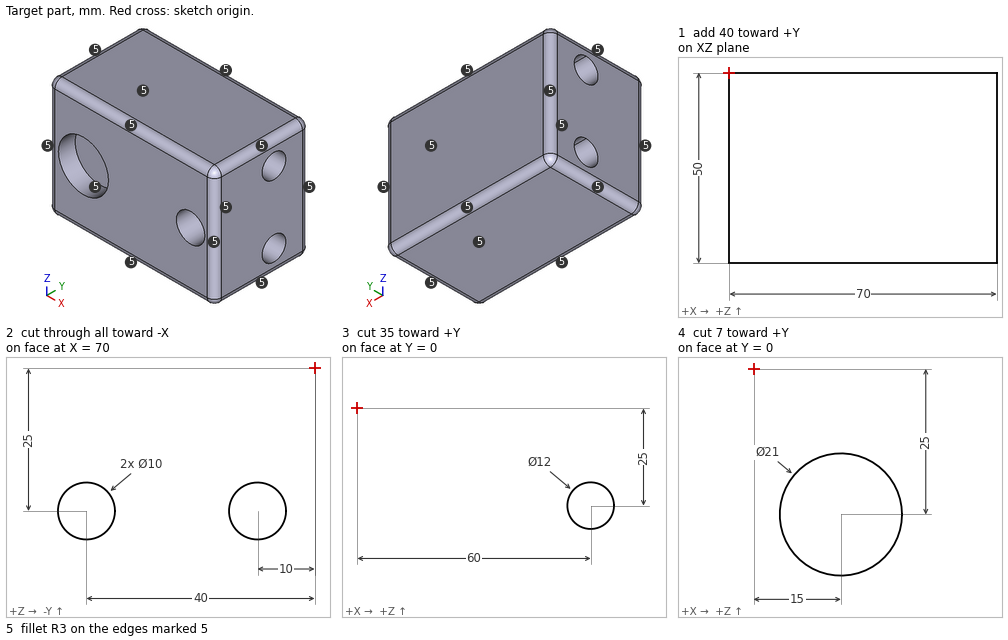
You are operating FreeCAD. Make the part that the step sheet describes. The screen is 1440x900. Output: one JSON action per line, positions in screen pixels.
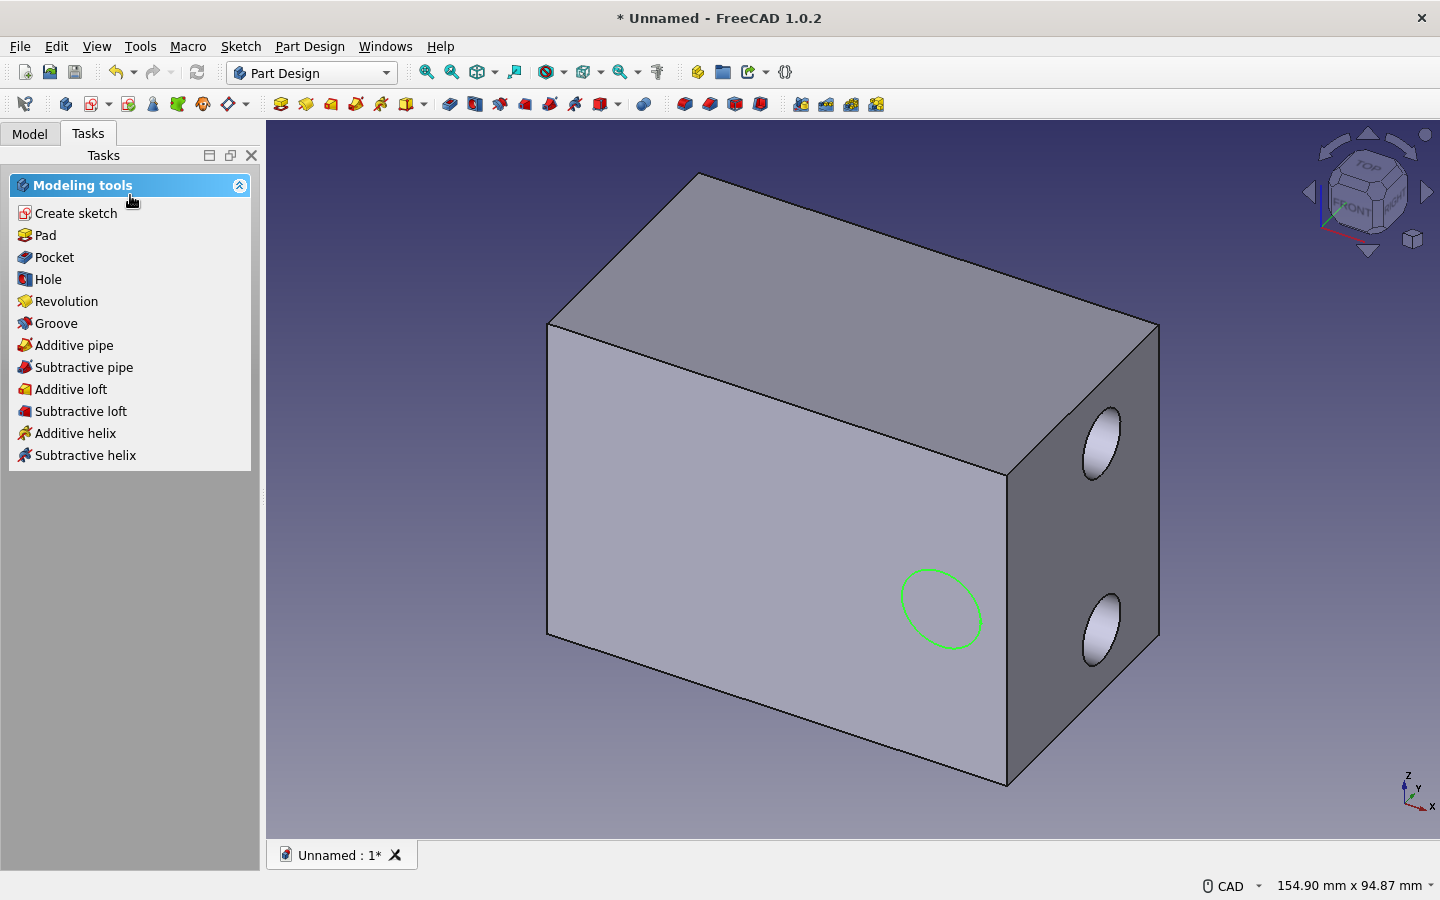
{"action": "left_click", "coordinate": [450, 104]}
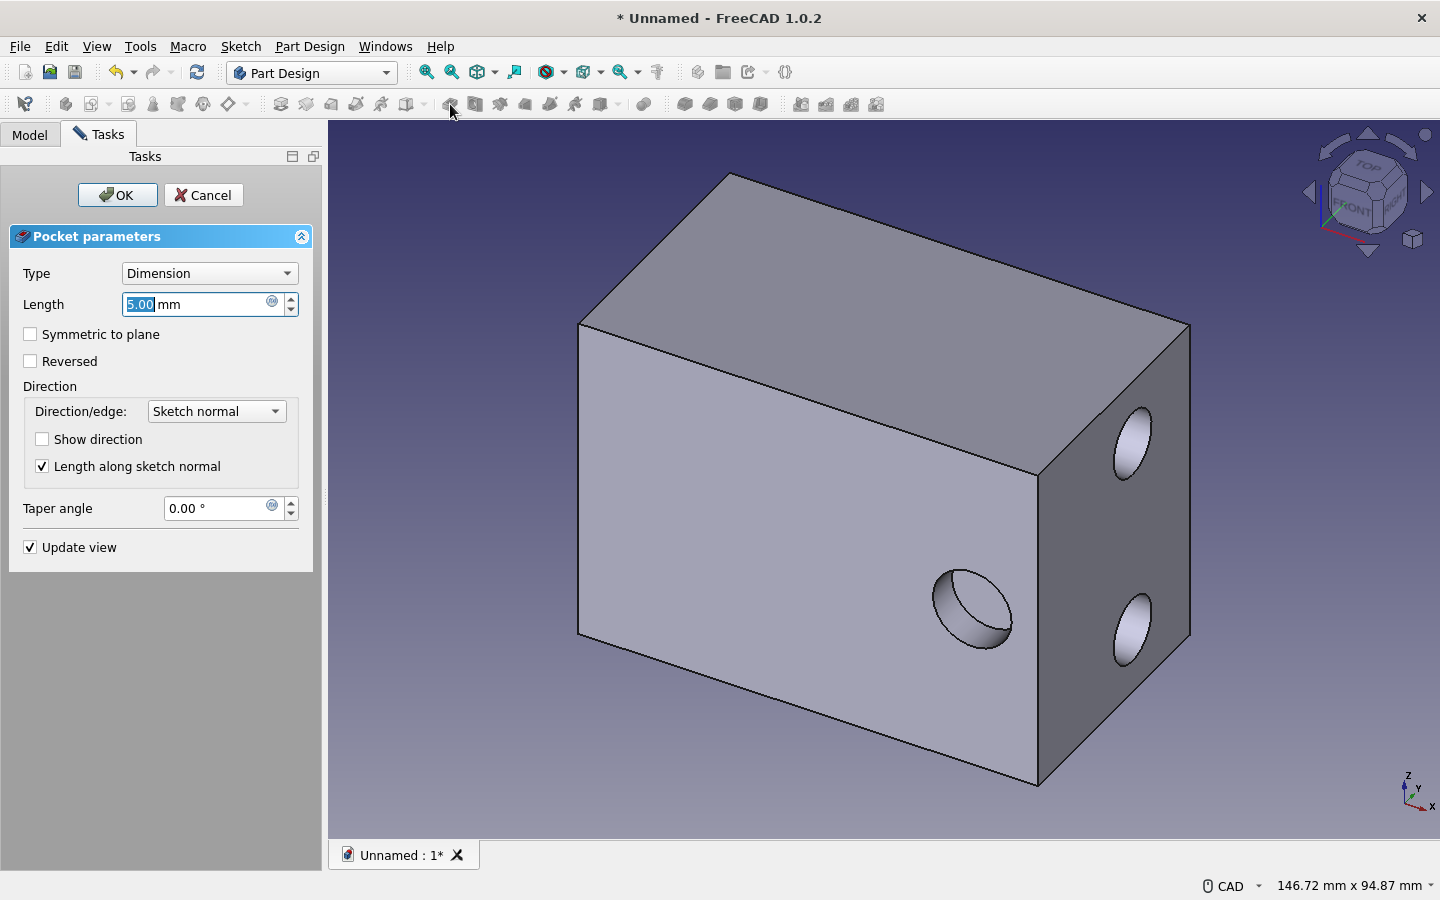
{"action": "type", "text": "35"}
{"action": "key", "text": "Tab"}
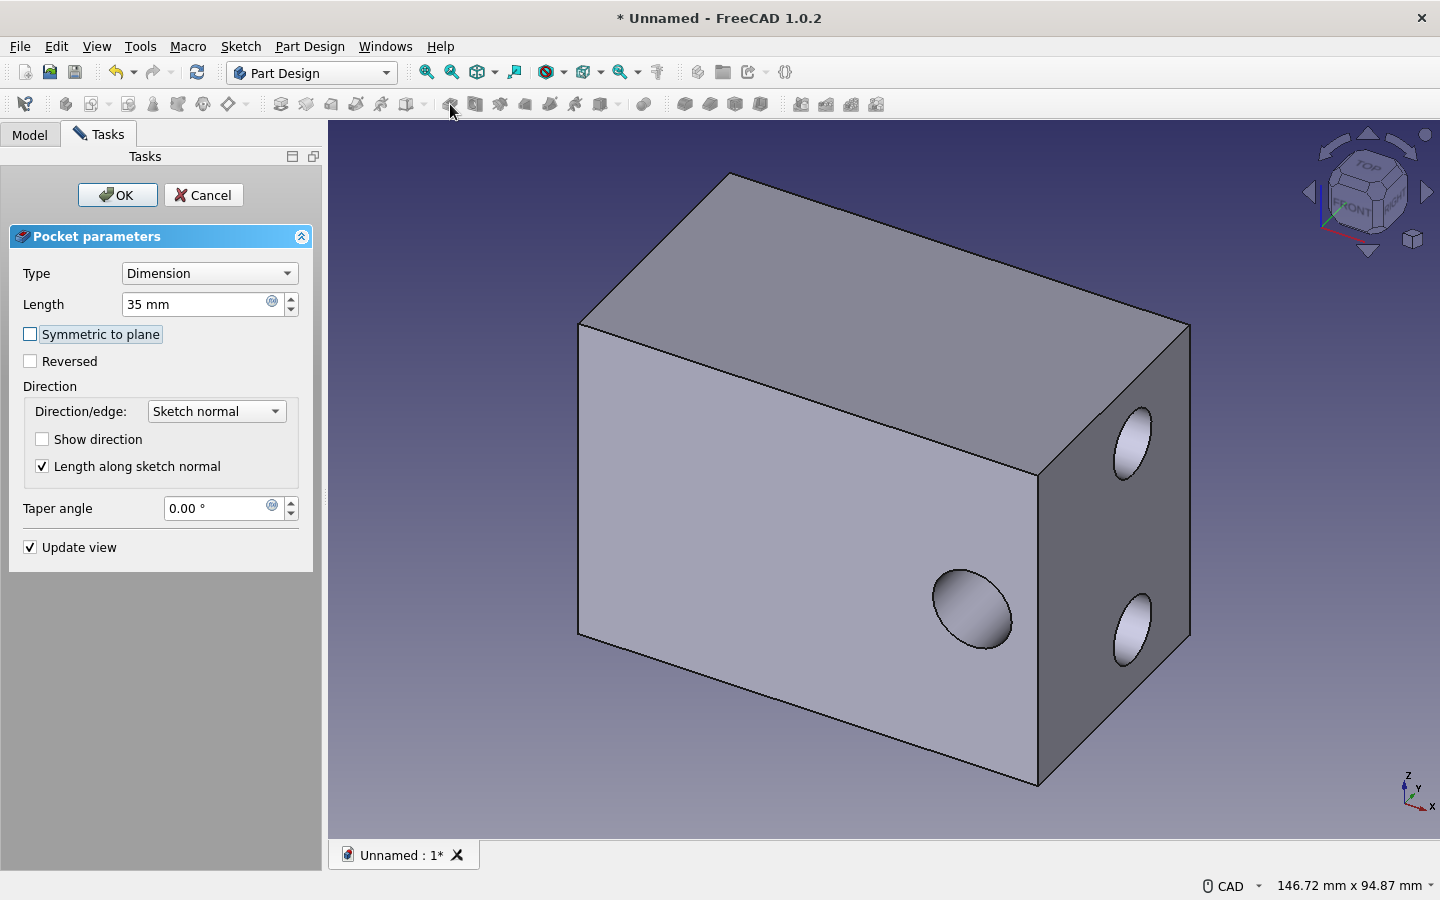
{"action": "left_click", "coordinate": [118, 195]}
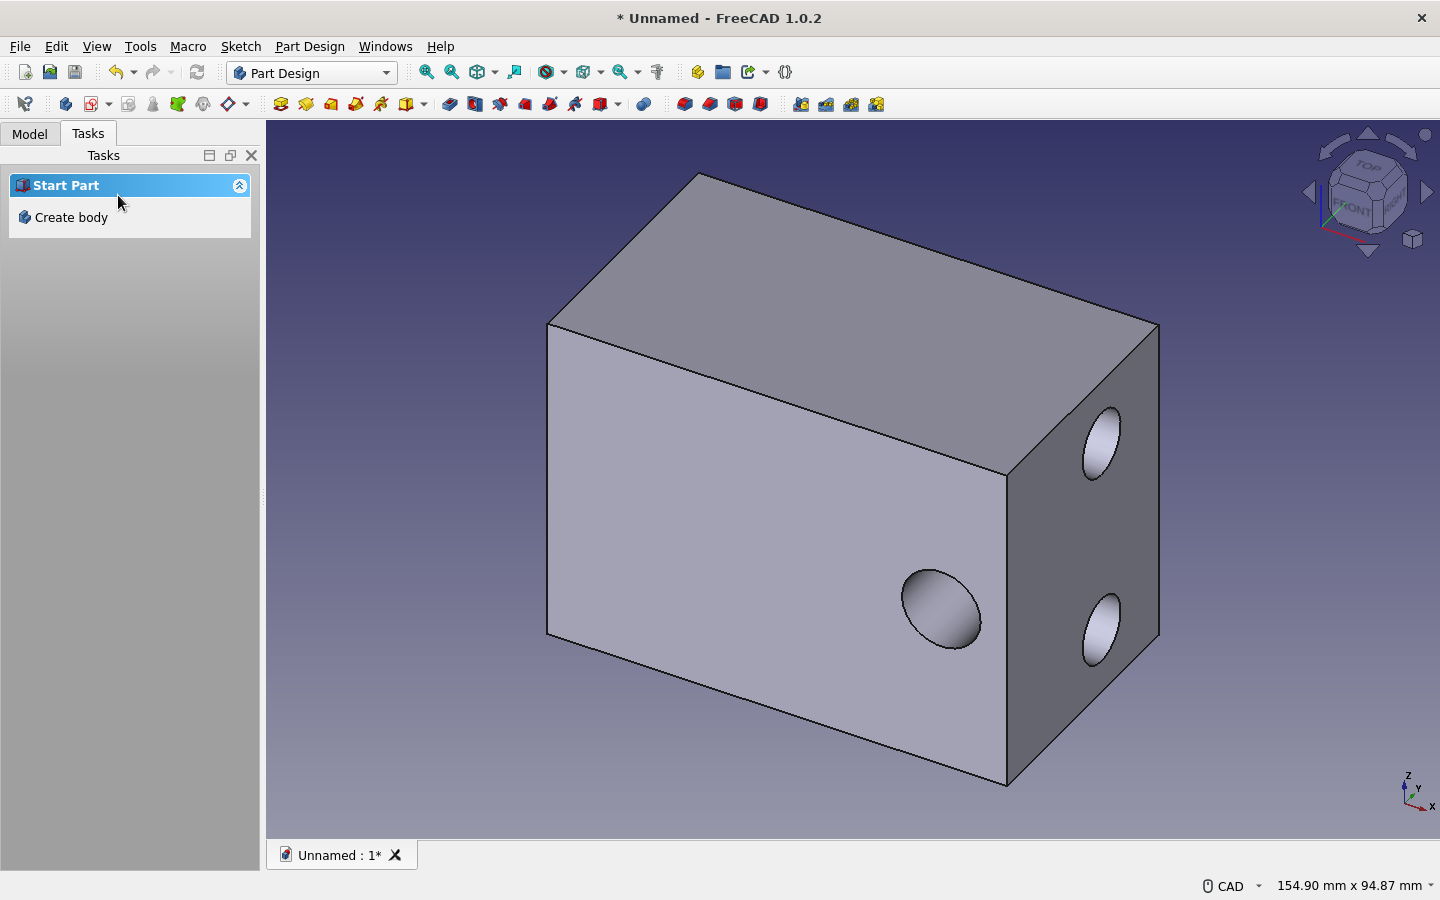
{"action": "left_click", "coordinate": [712, 532]}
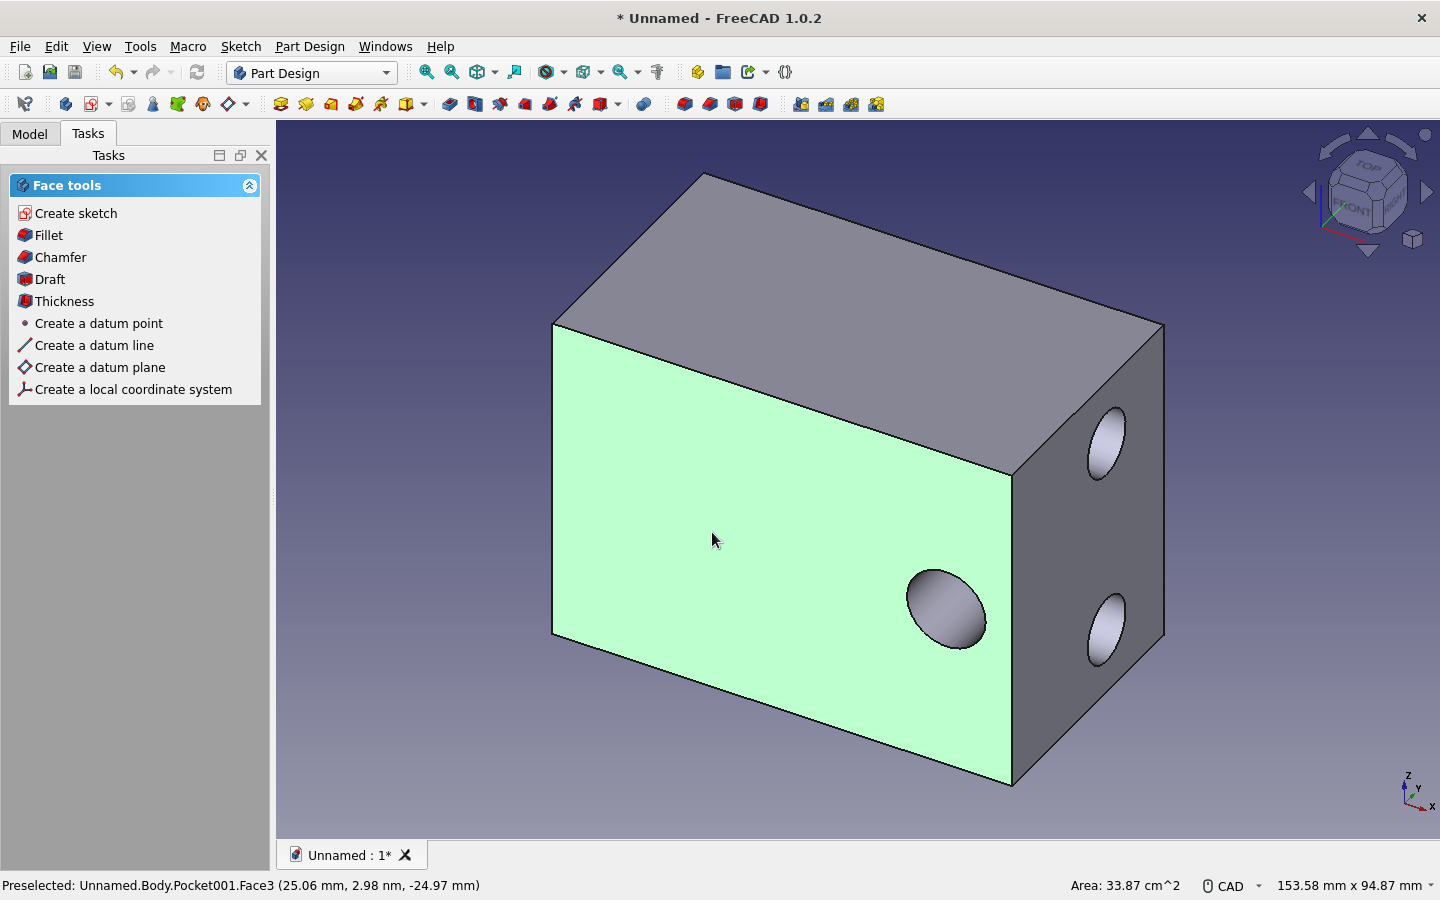
{"action": "left_click", "coordinate": [90, 104]}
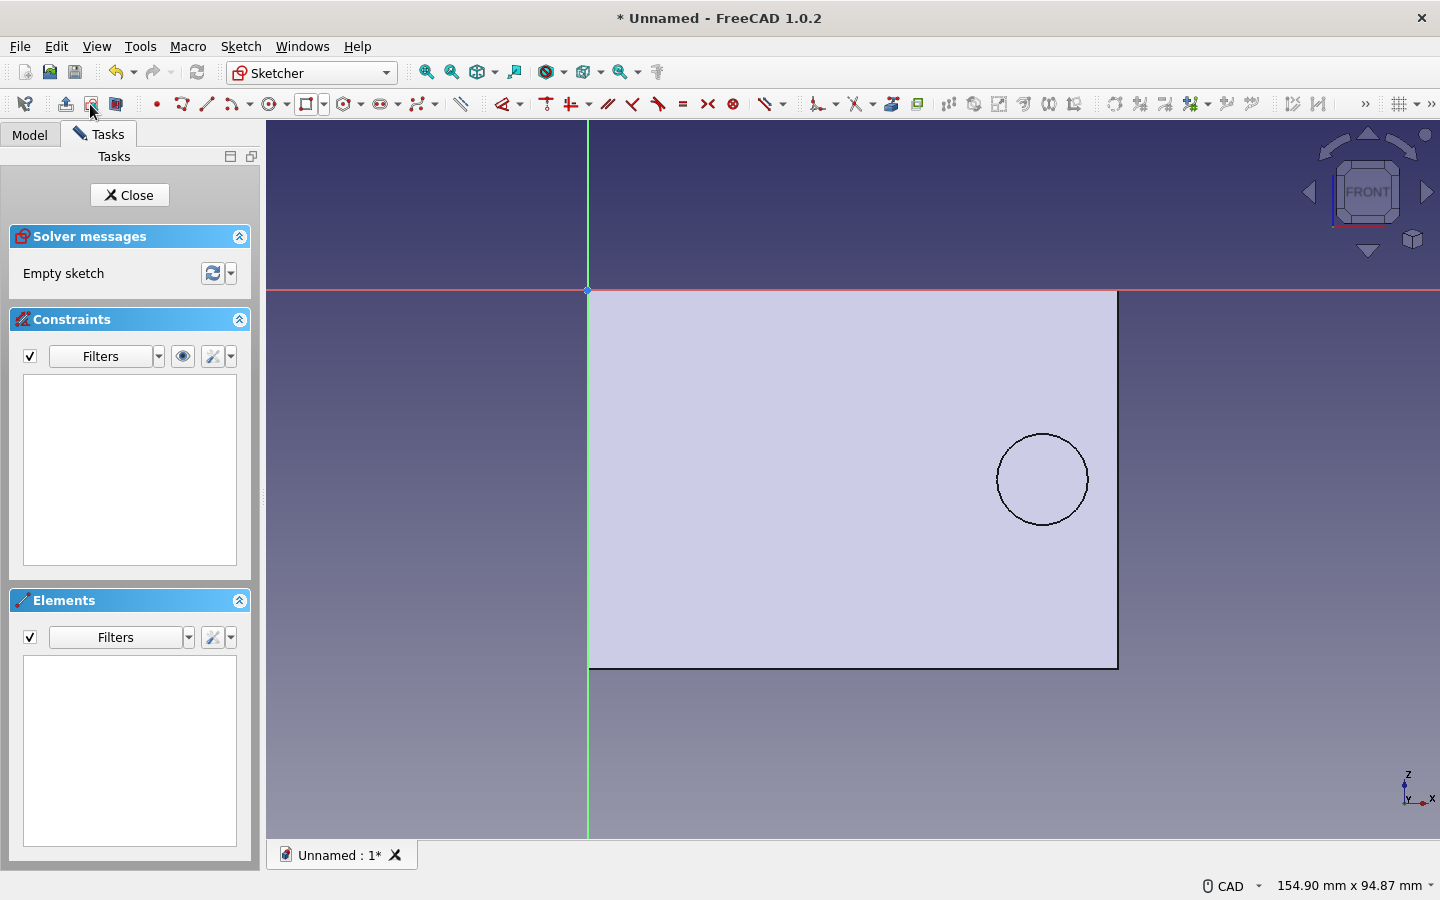
{"action": "scroll", "coordinate": [563, 358], "scroll_direction": "up", "scroll_amount": 3}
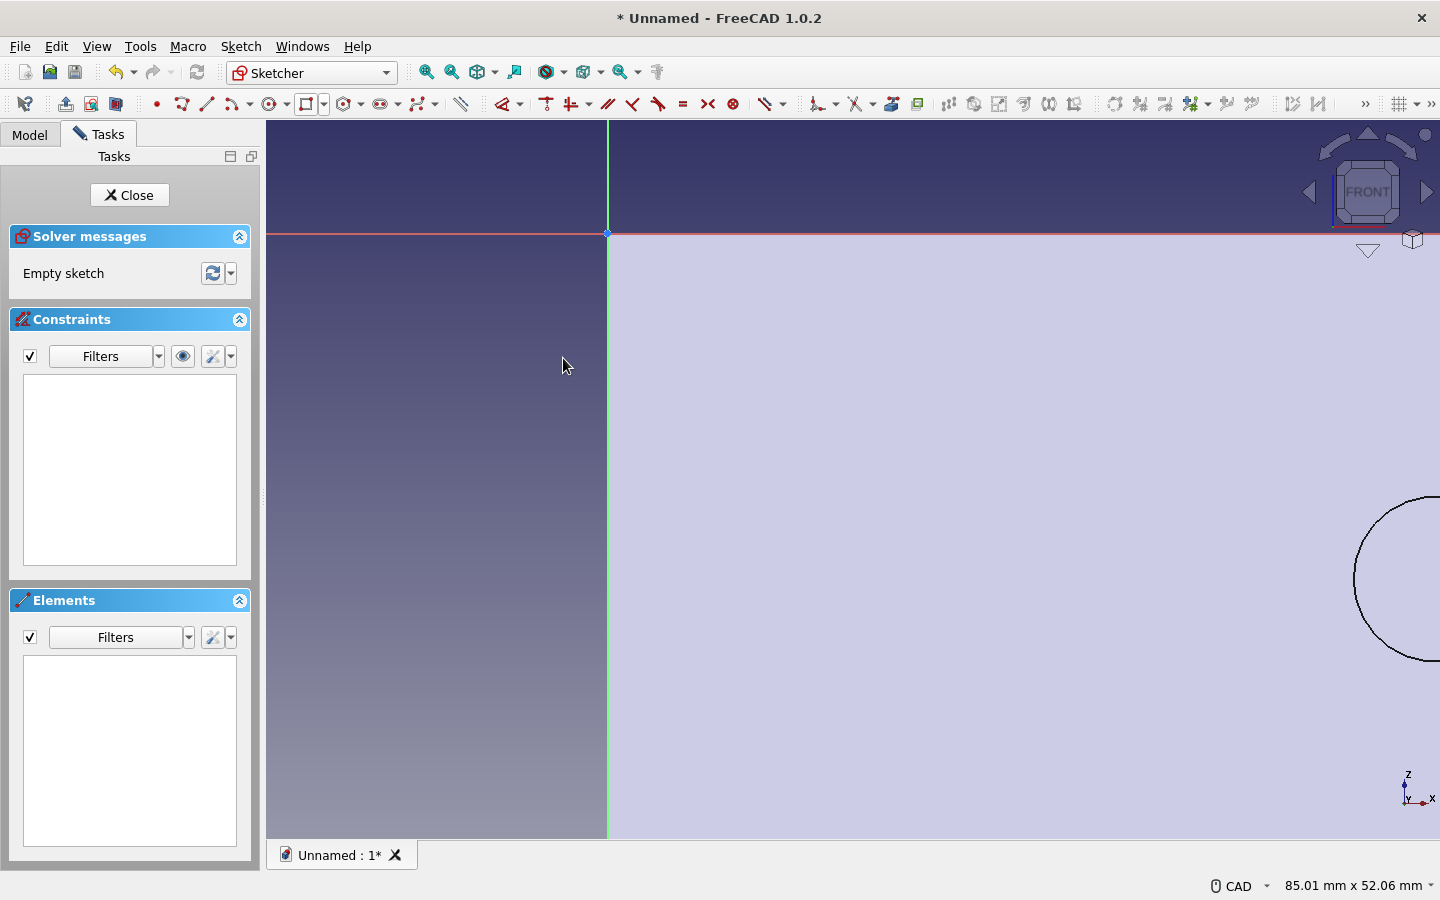
{"action": "left_click", "coordinate": [268, 104]}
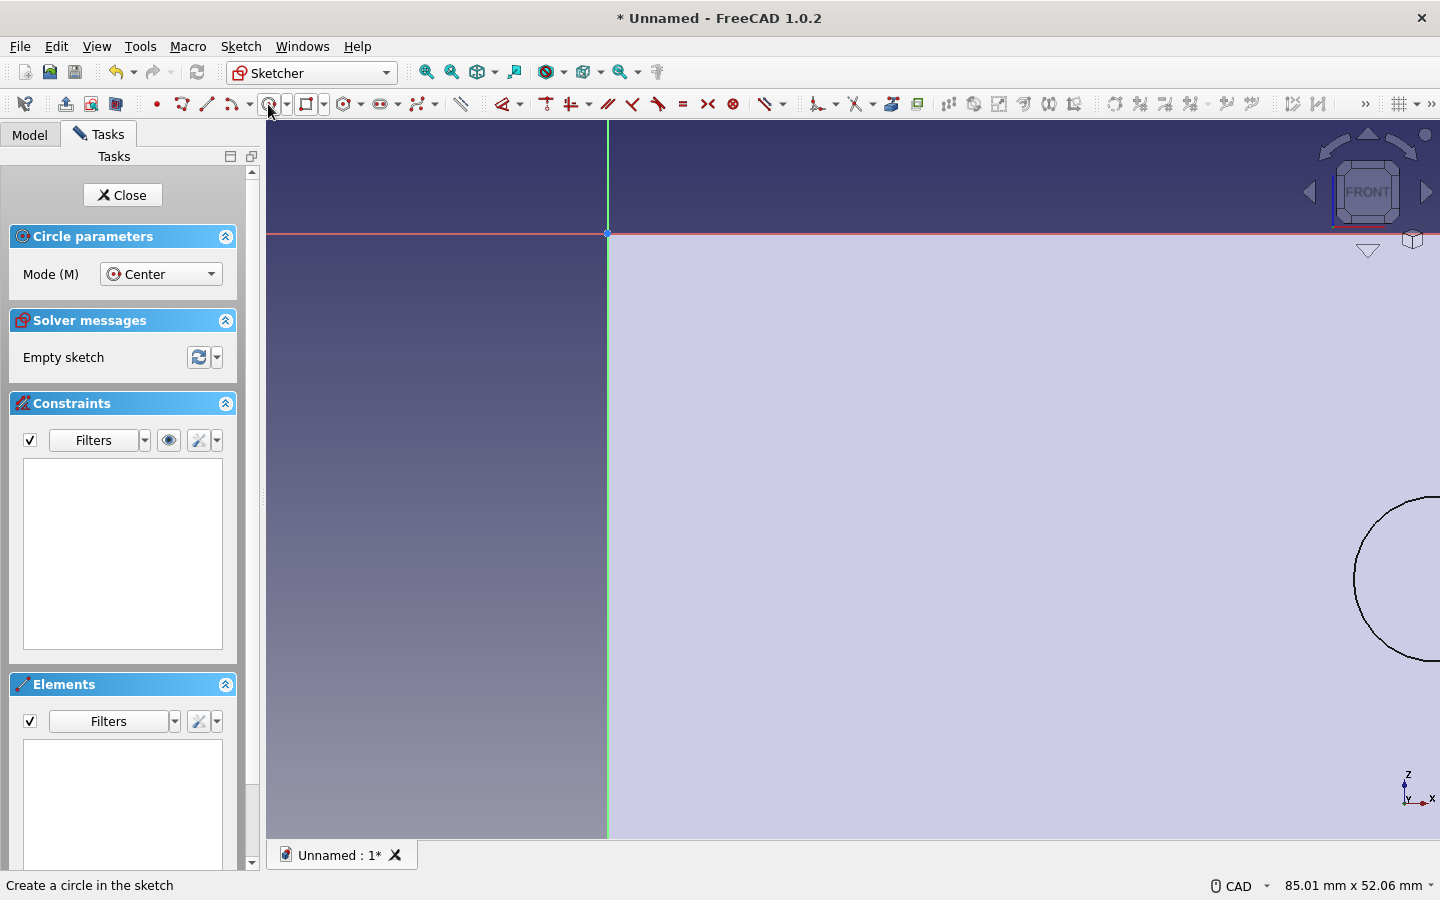
{"action": "left_click", "coordinate": [815, 579]}
{"action": "left_click", "coordinate": [918, 477]}
{"action": "key", "text": "Escape"}